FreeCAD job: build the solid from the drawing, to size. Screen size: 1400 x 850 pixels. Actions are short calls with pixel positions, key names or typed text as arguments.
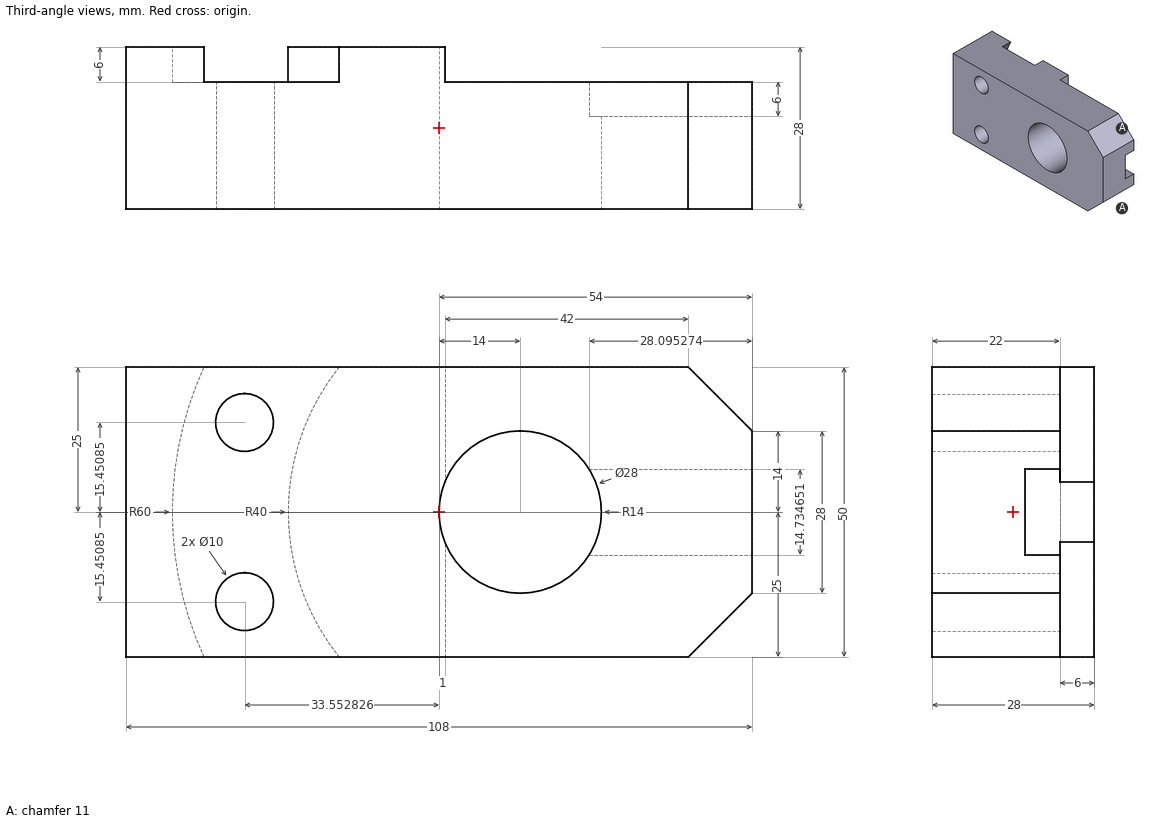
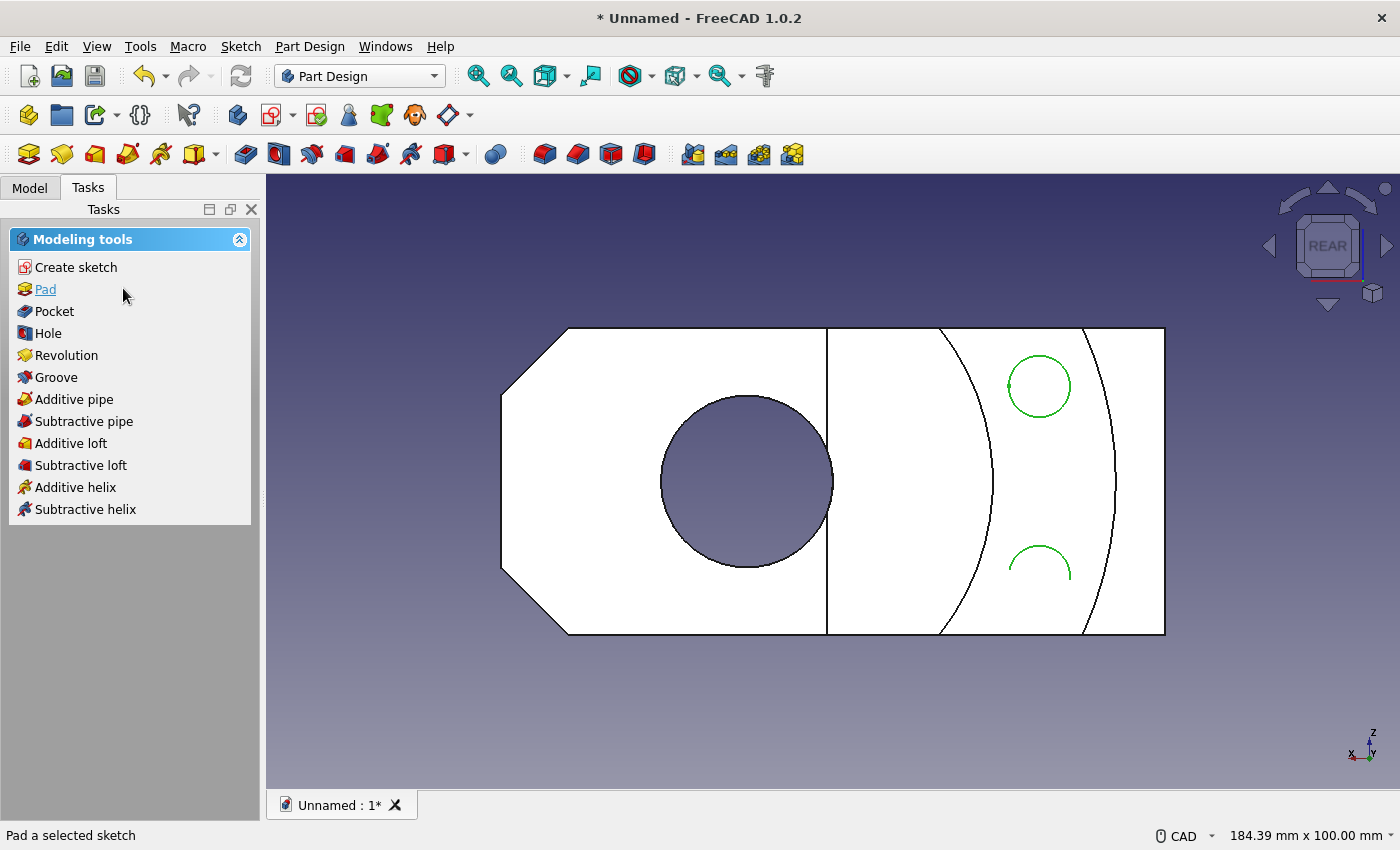
click(246, 154)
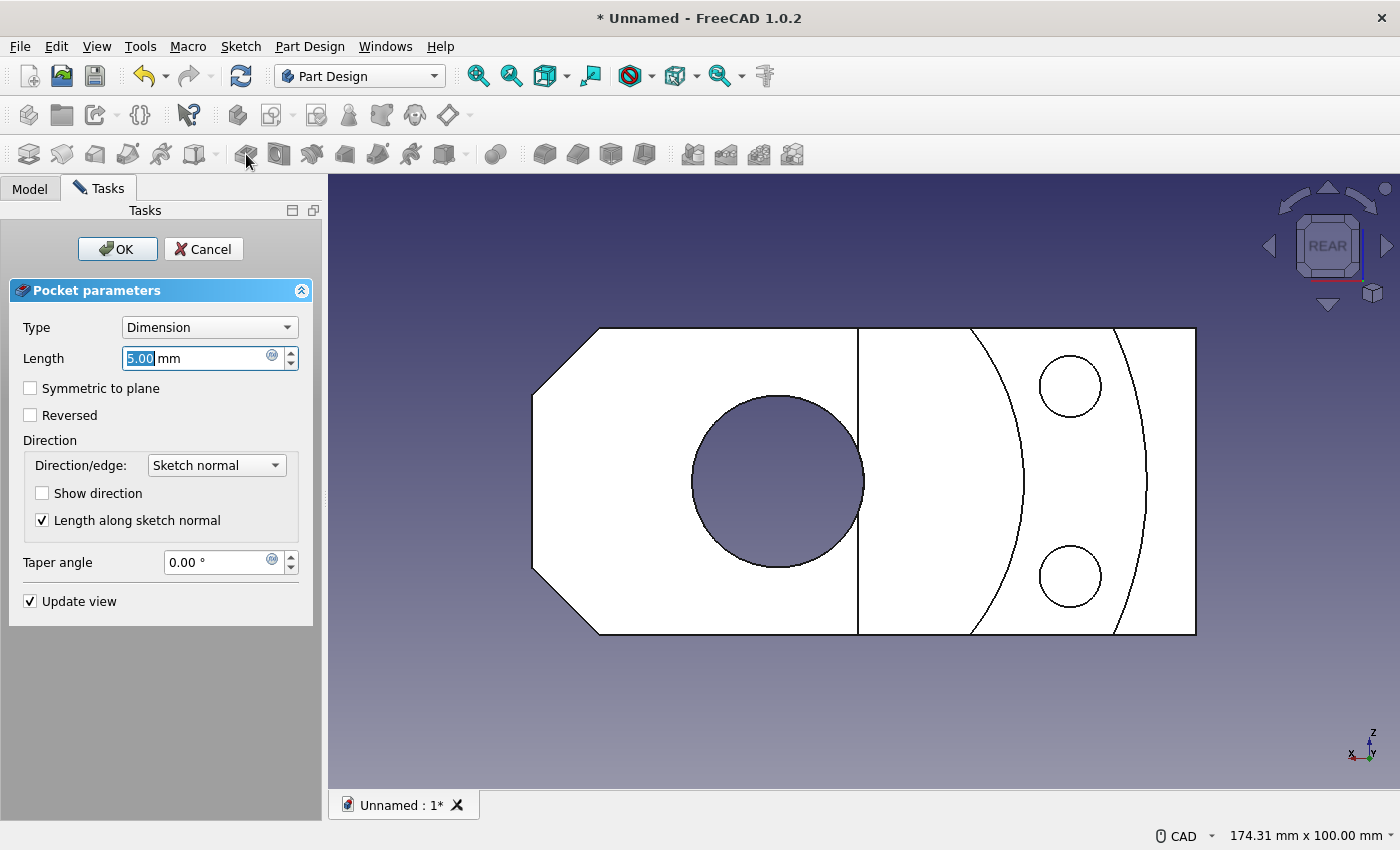
text(22)
key(Tab)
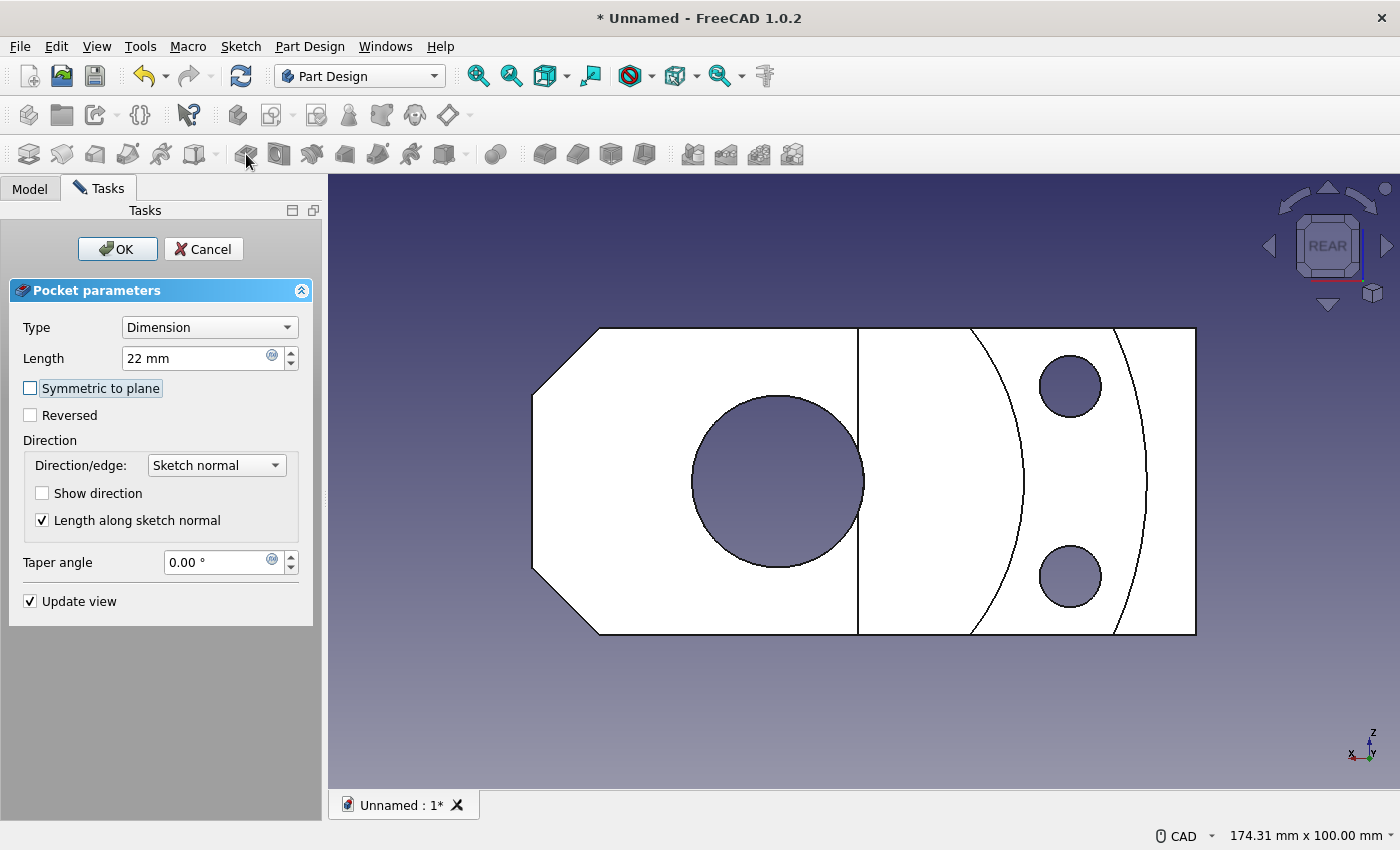
click(118, 249)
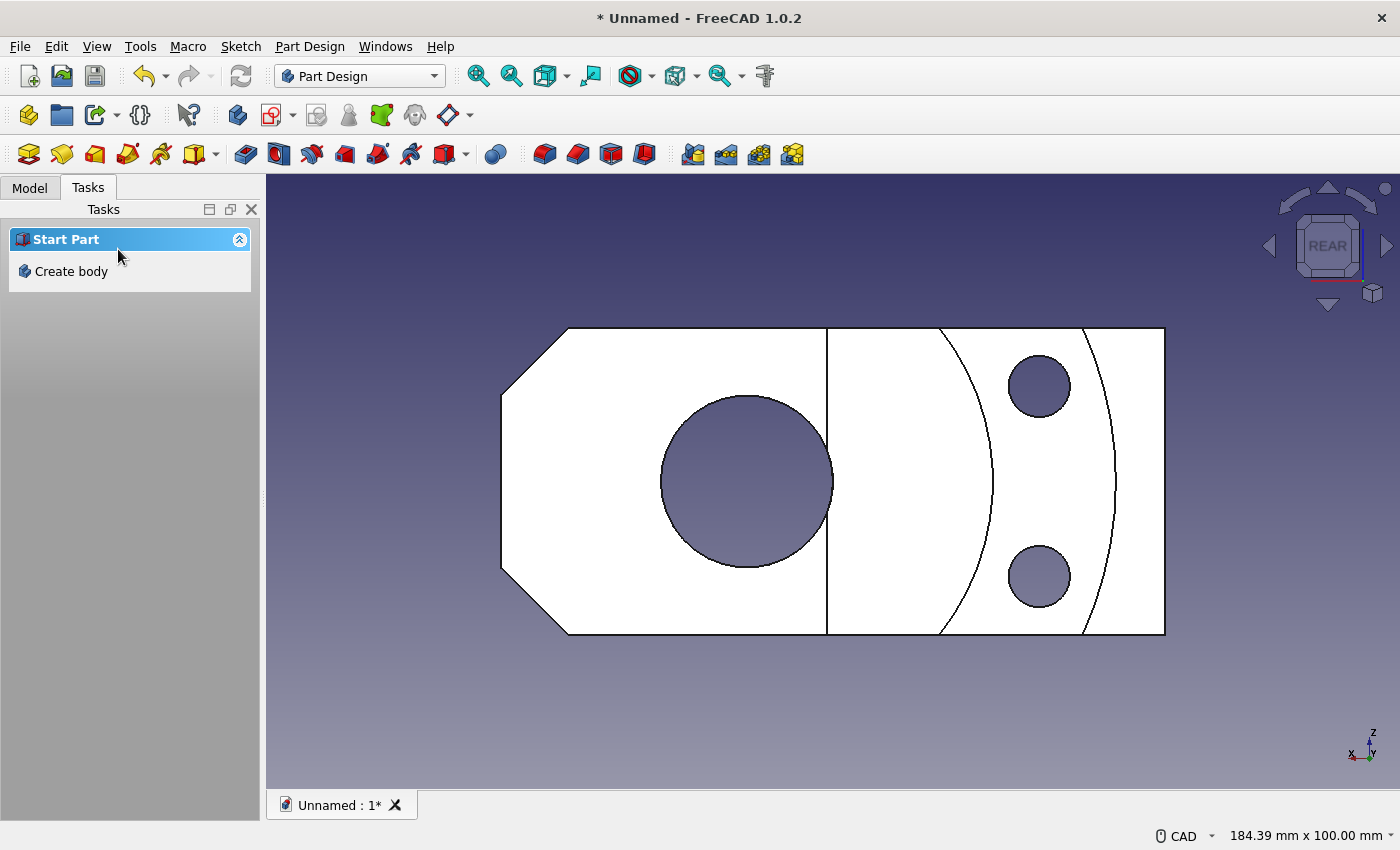
click(571, 437)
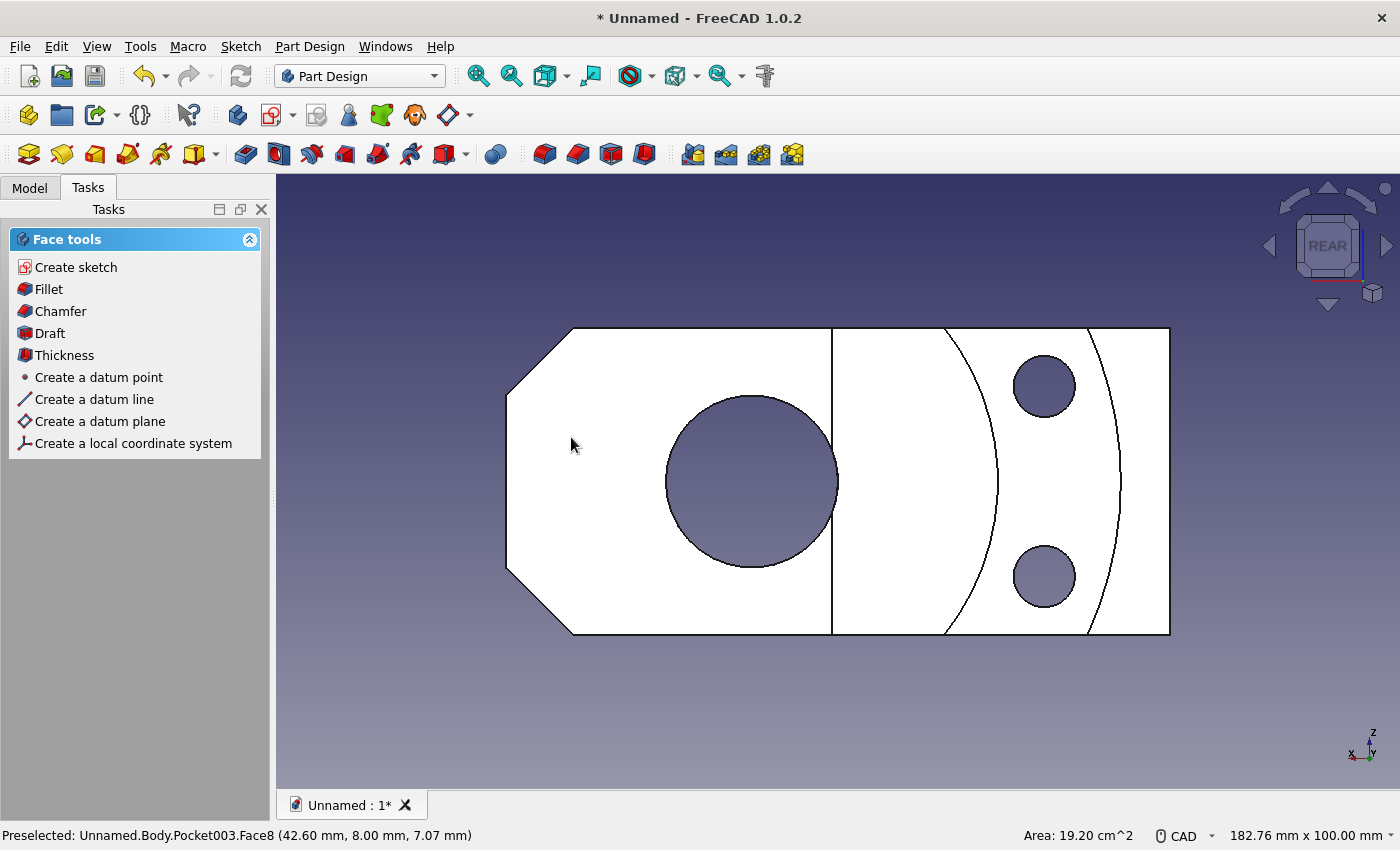
click(270, 116)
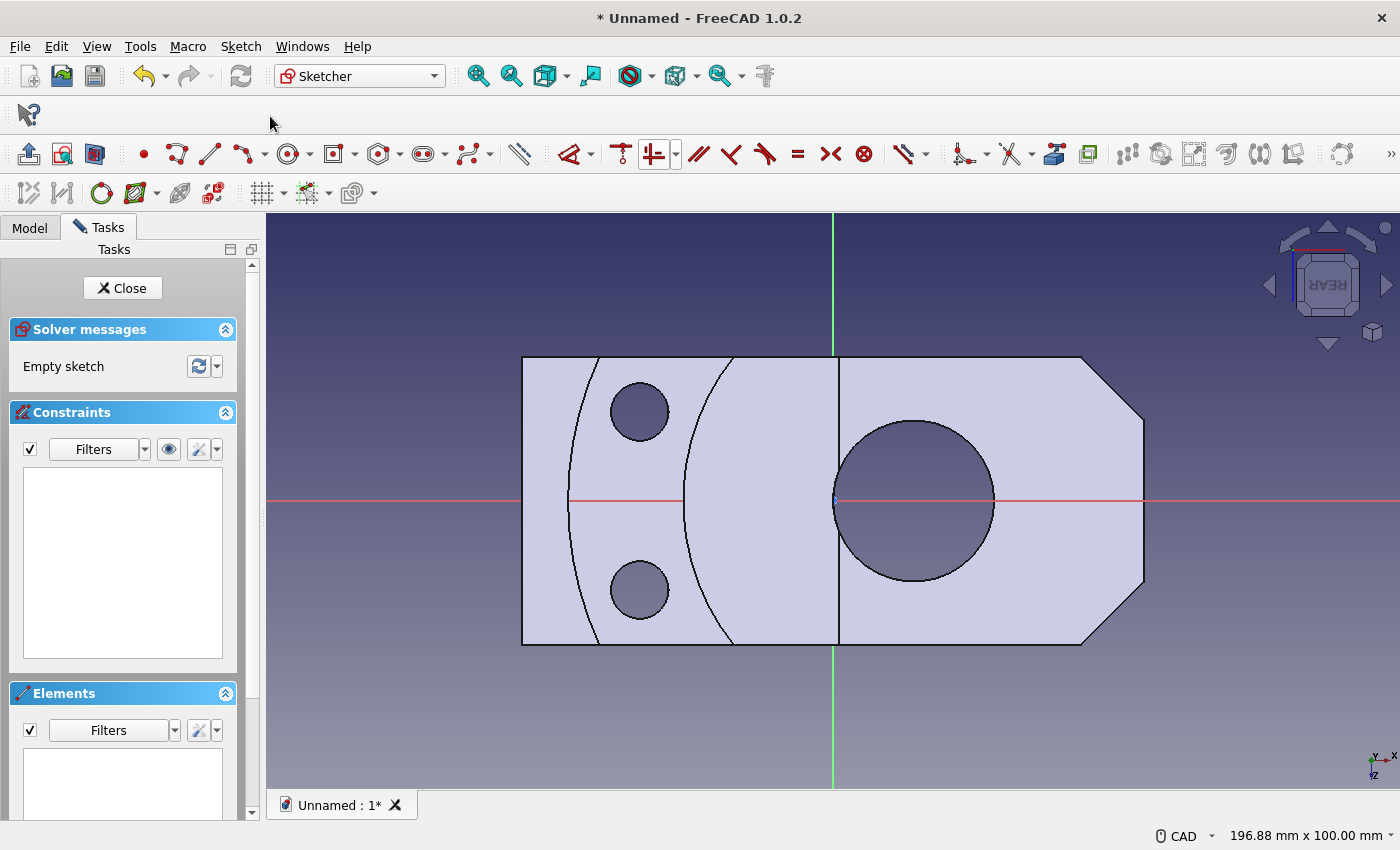
key(q)
key(s)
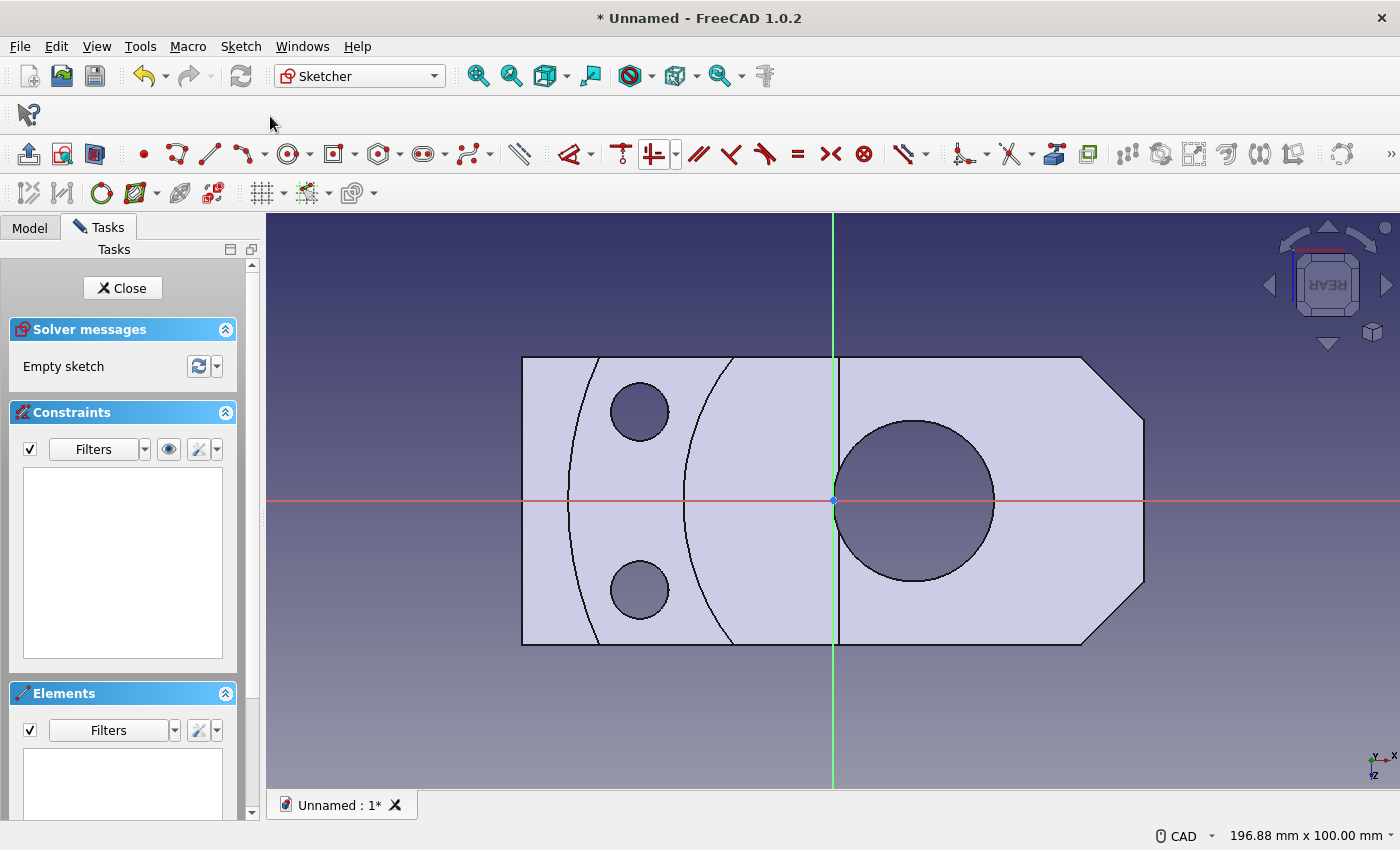
scroll(1171, 501, up, 4)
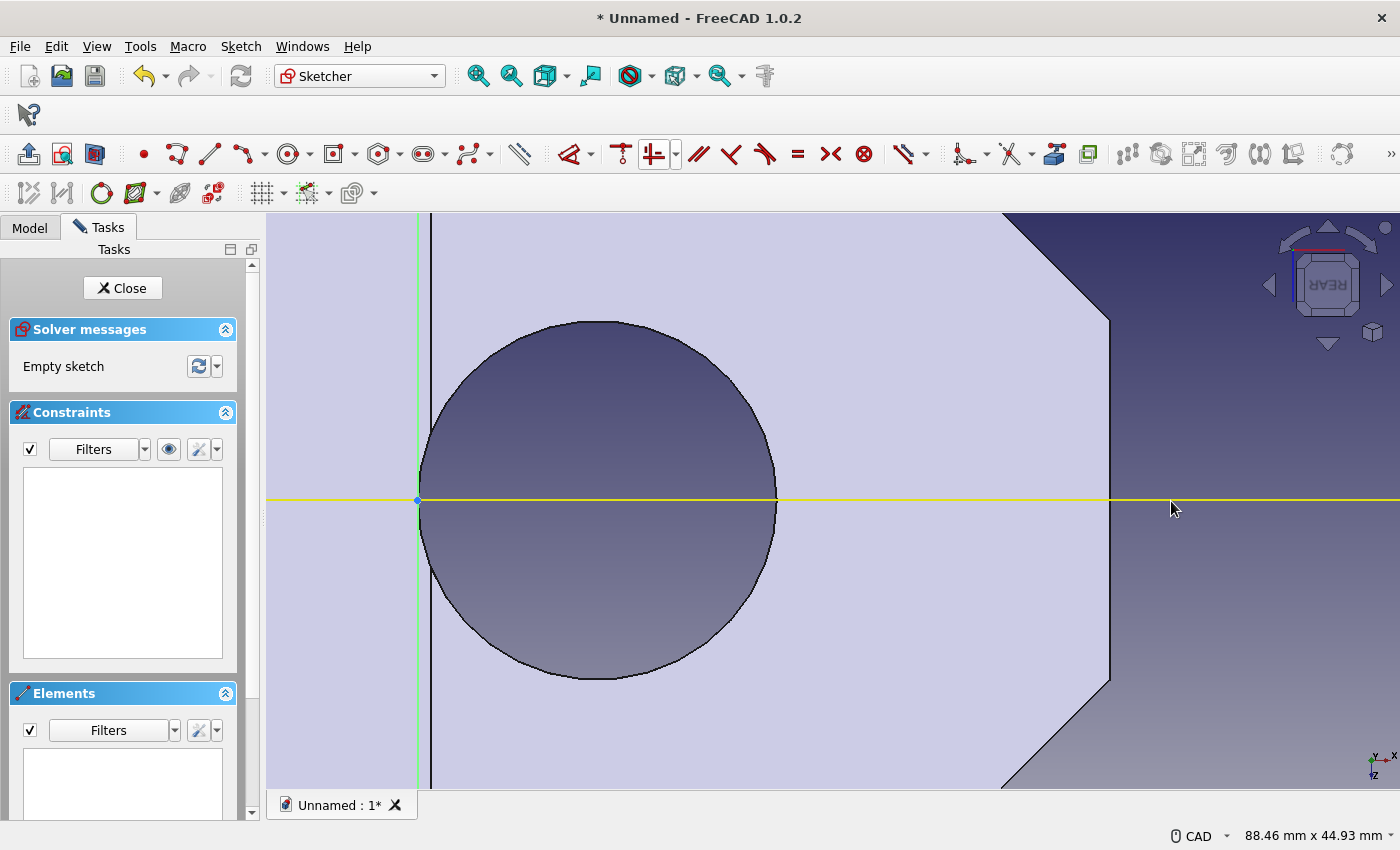
click(177, 154)